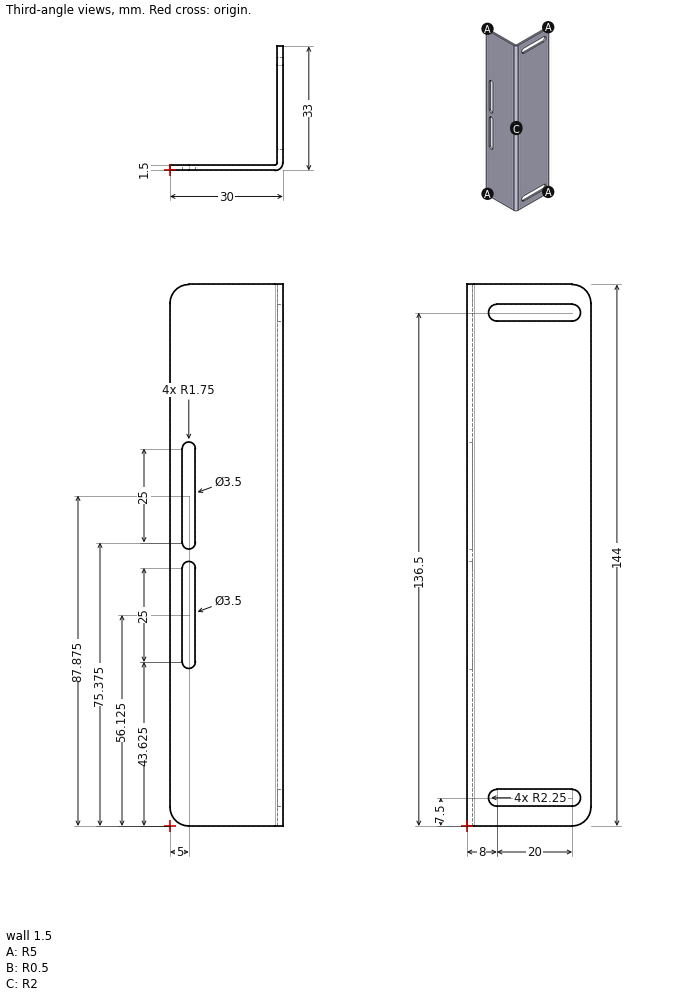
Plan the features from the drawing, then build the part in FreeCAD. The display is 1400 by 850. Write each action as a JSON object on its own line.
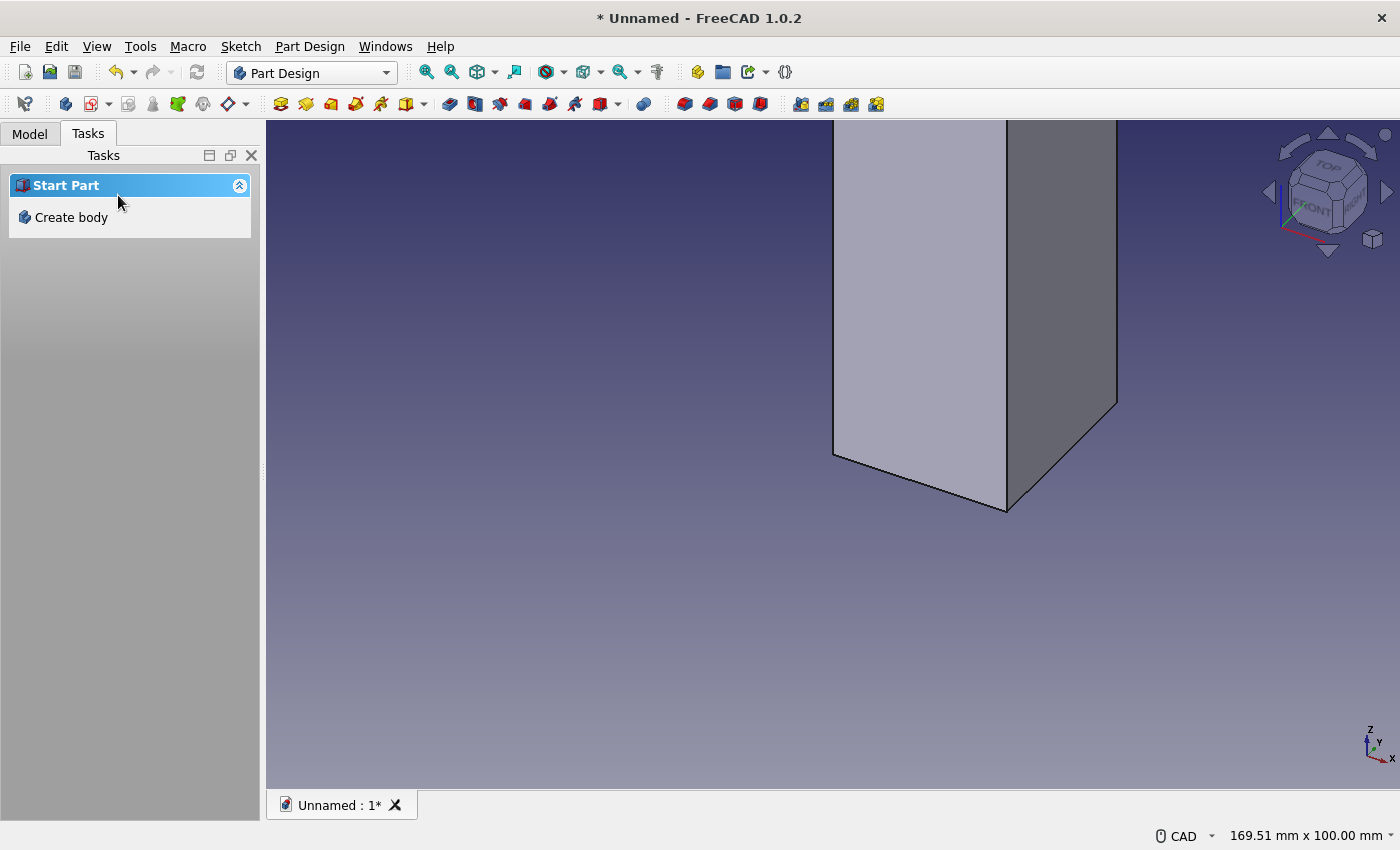
{"action": "left_click", "coordinate": [427, 72]}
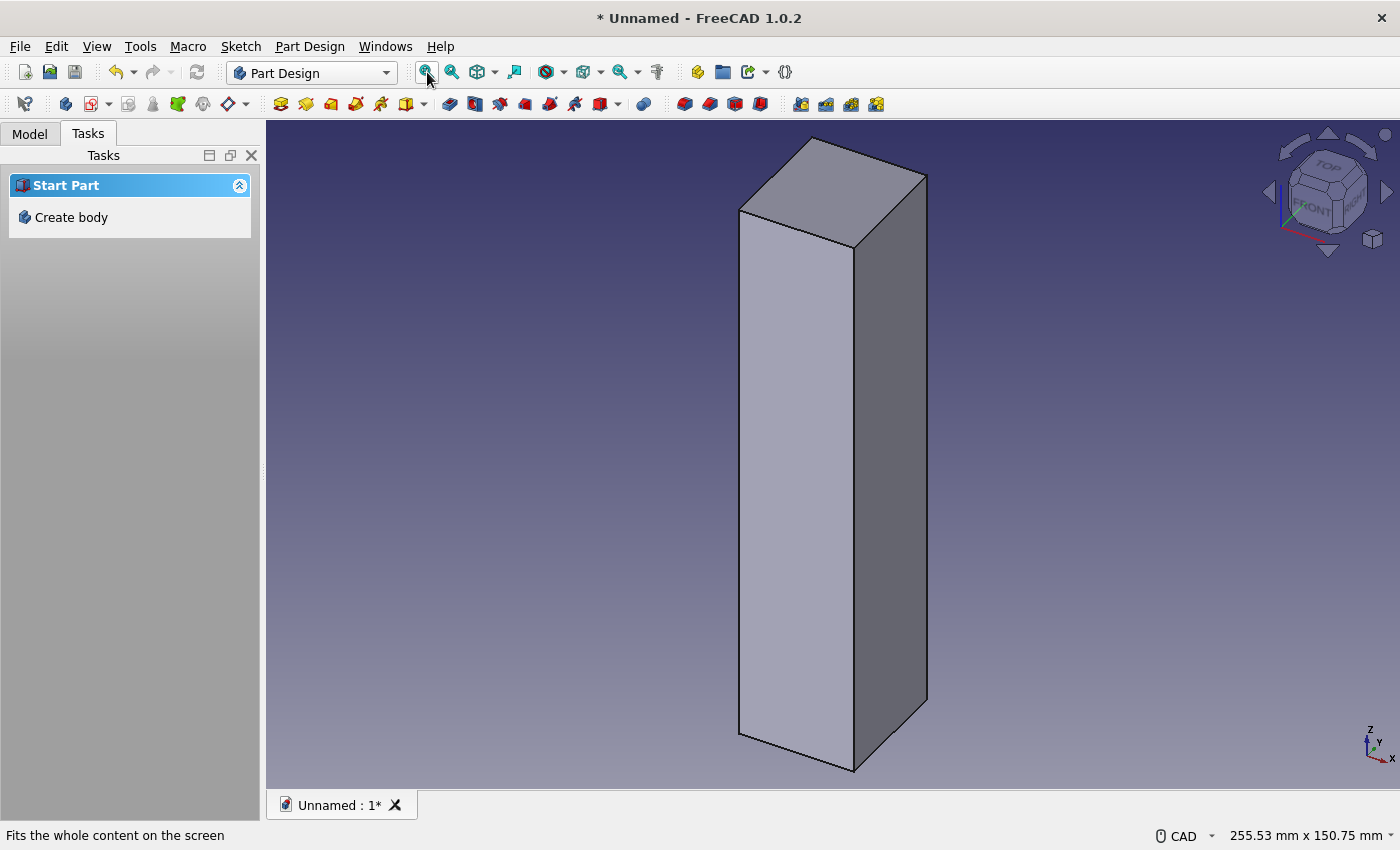
{"action": "left_click", "coordinate": [833, 192]}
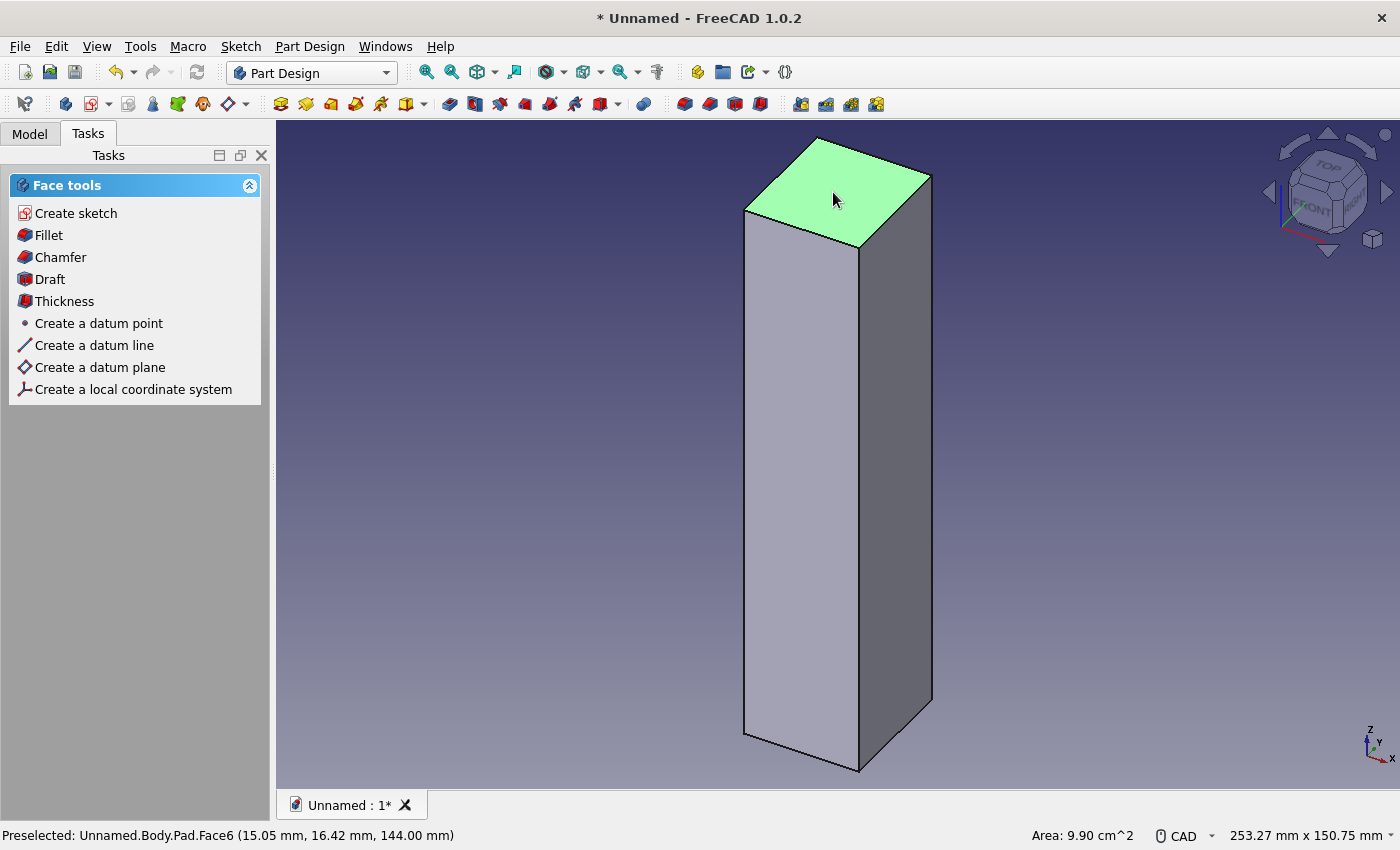
{"action": "key", "text": "0"}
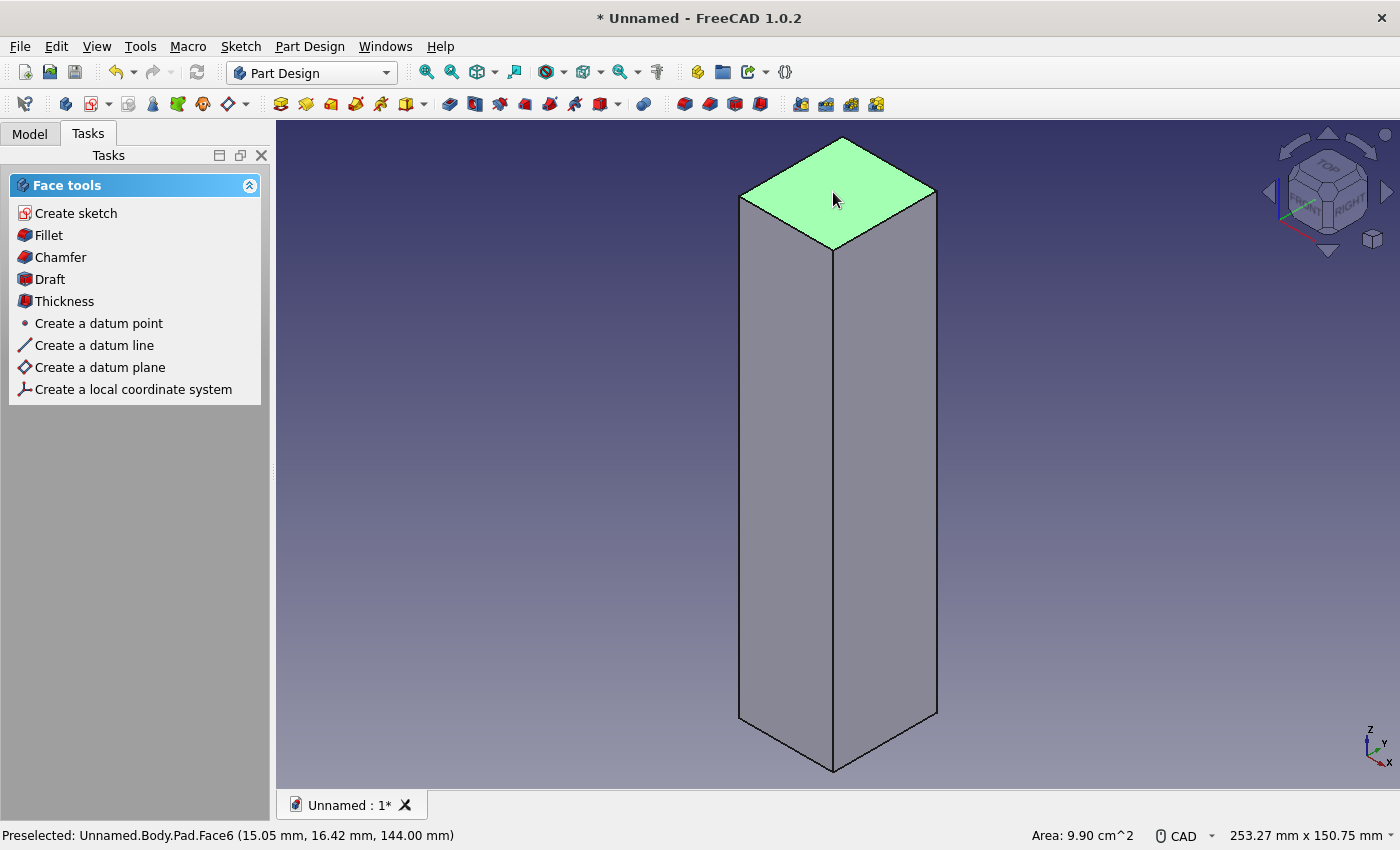
{"action": "key", "text": "2"}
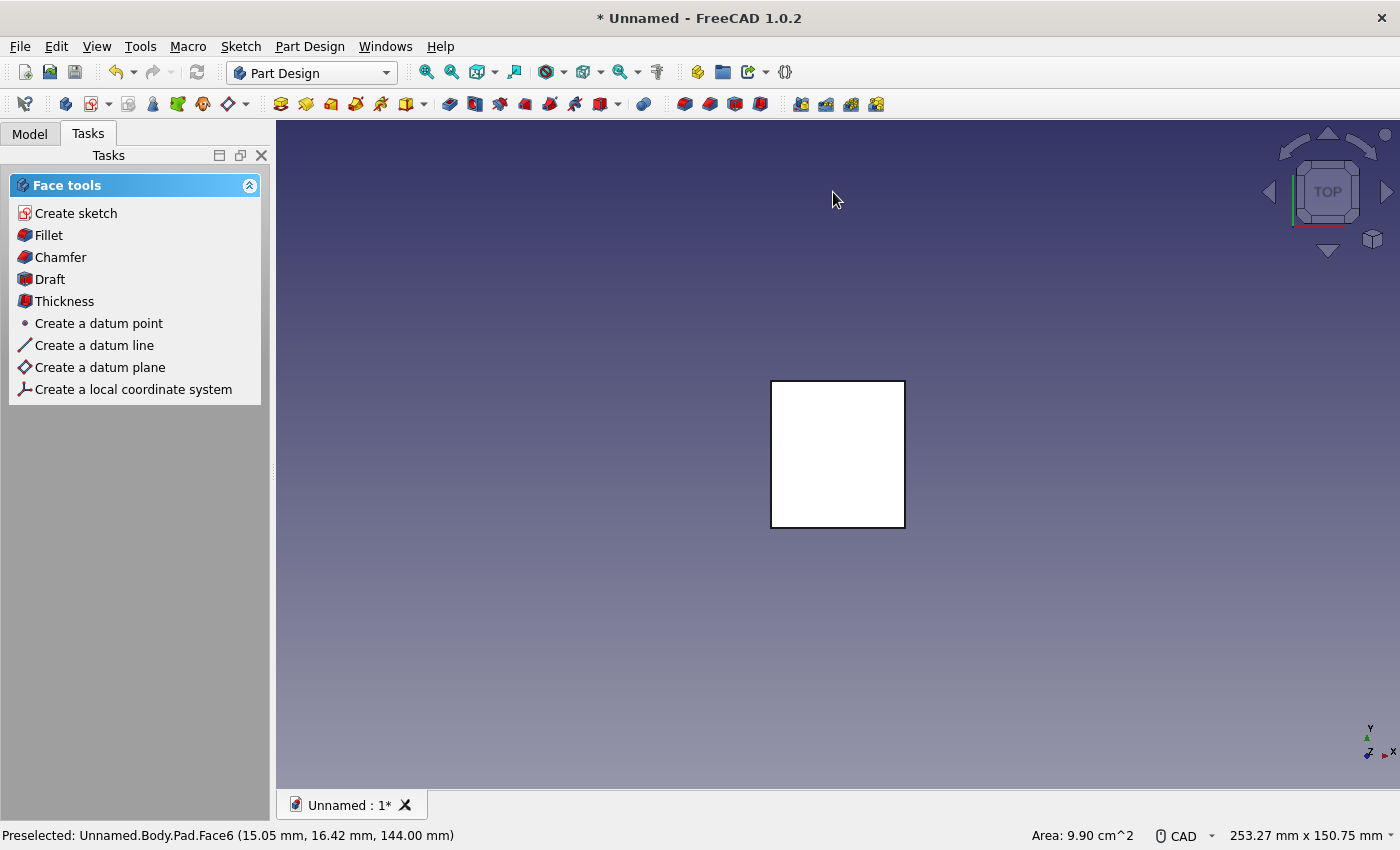
{"action": "left_click", "coordinate": [427, 72]}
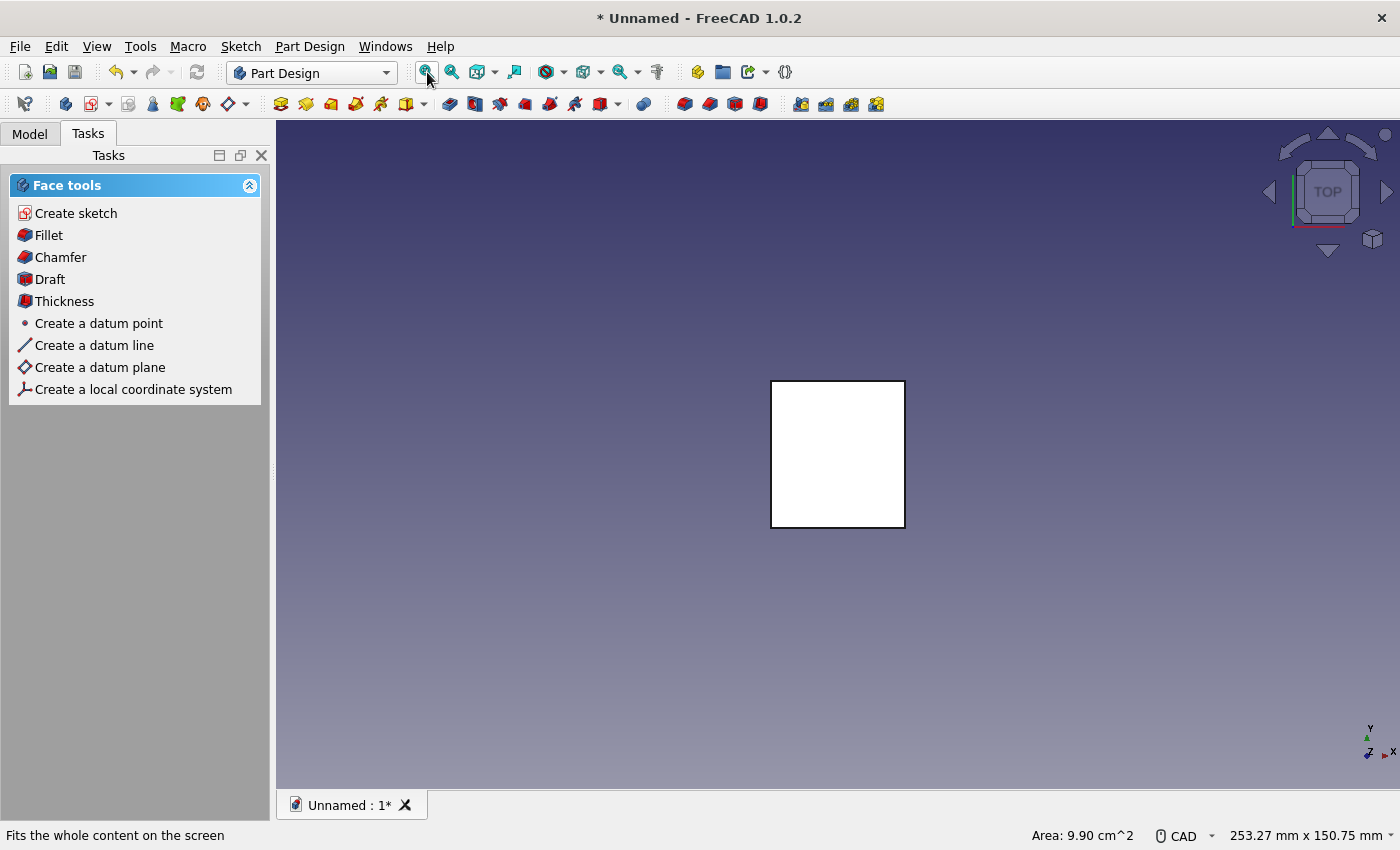
{"action": "key", "text": "1"}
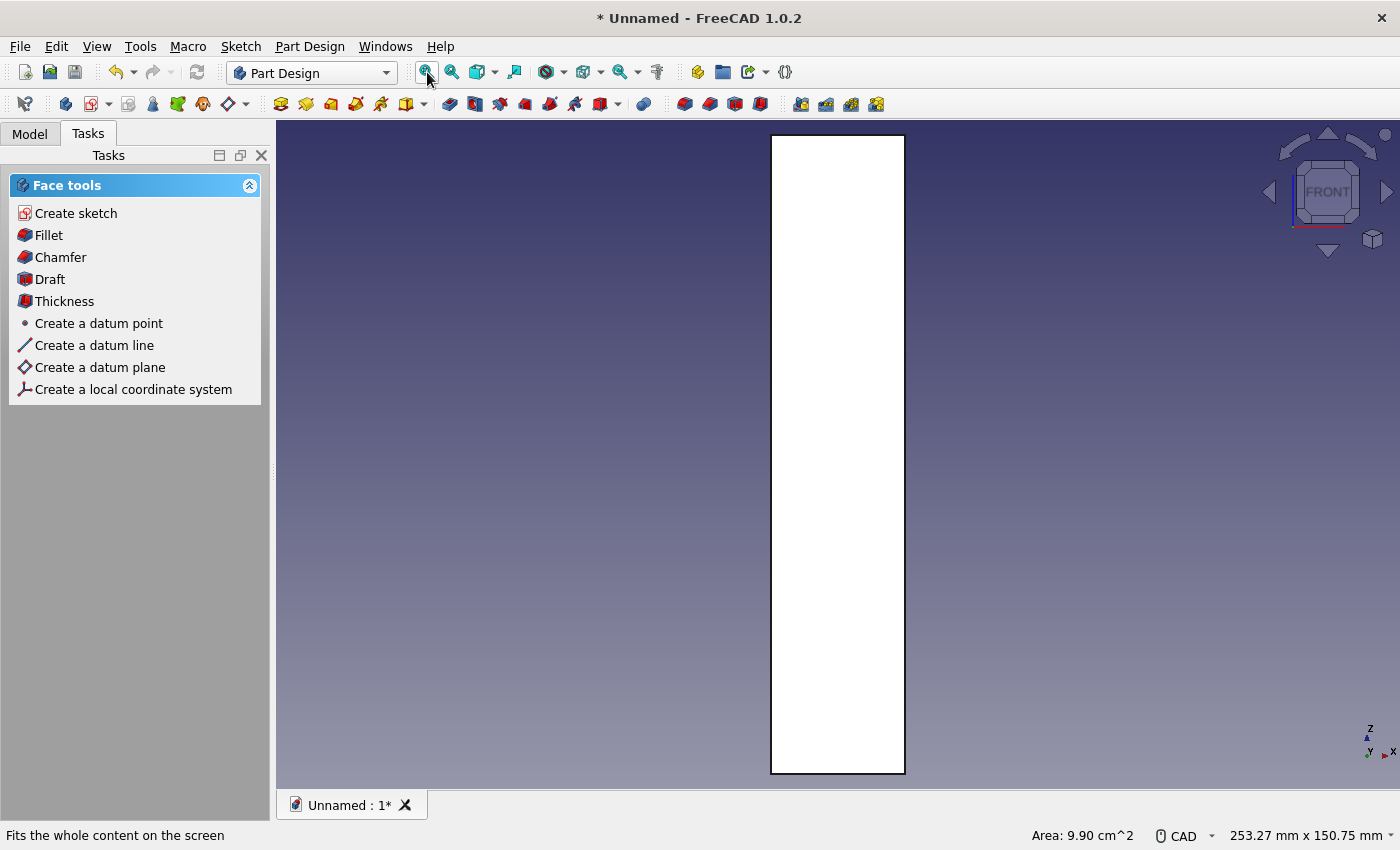
{"action": "key", "text": "3"}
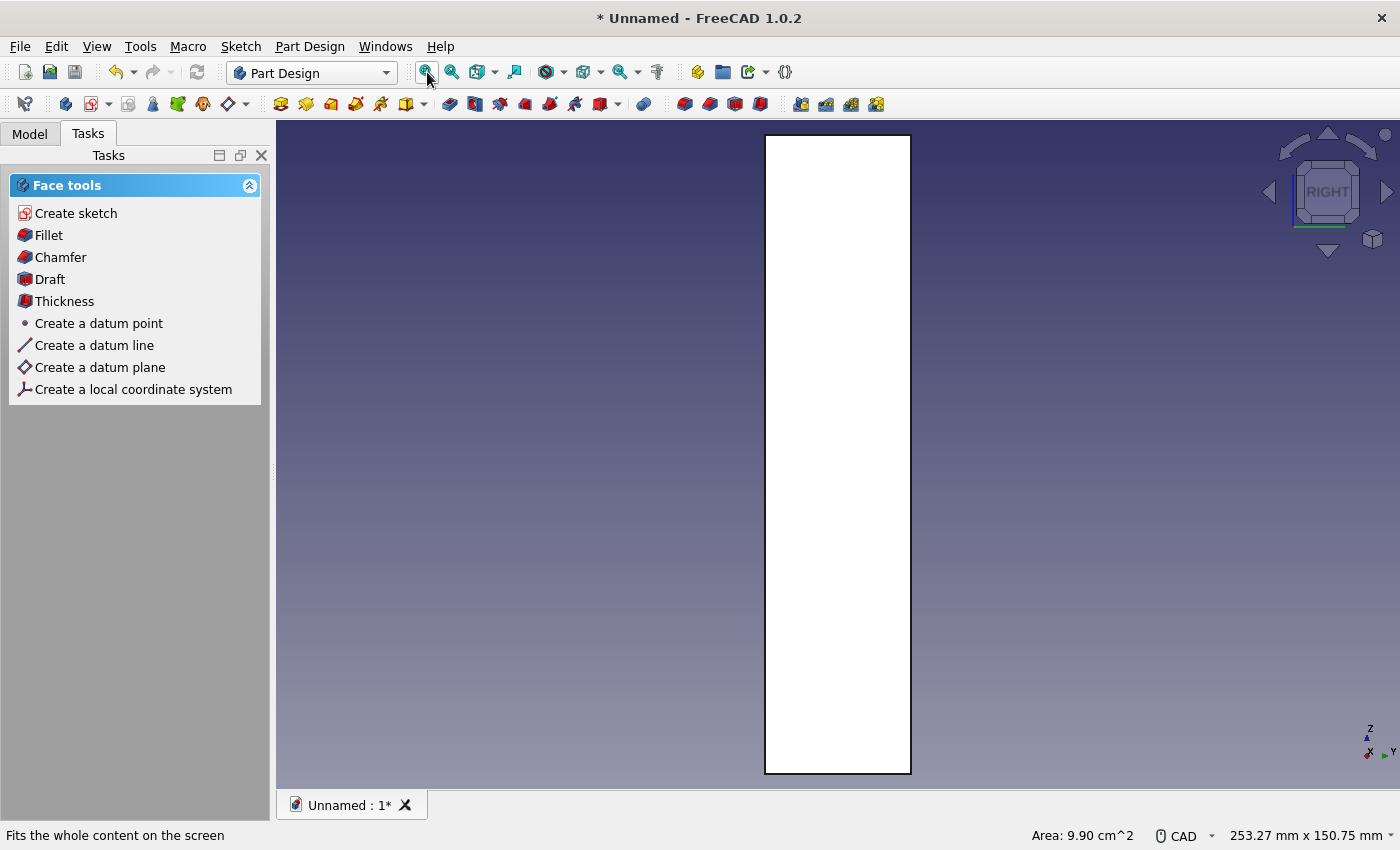
{"action": "key", "text": "5"}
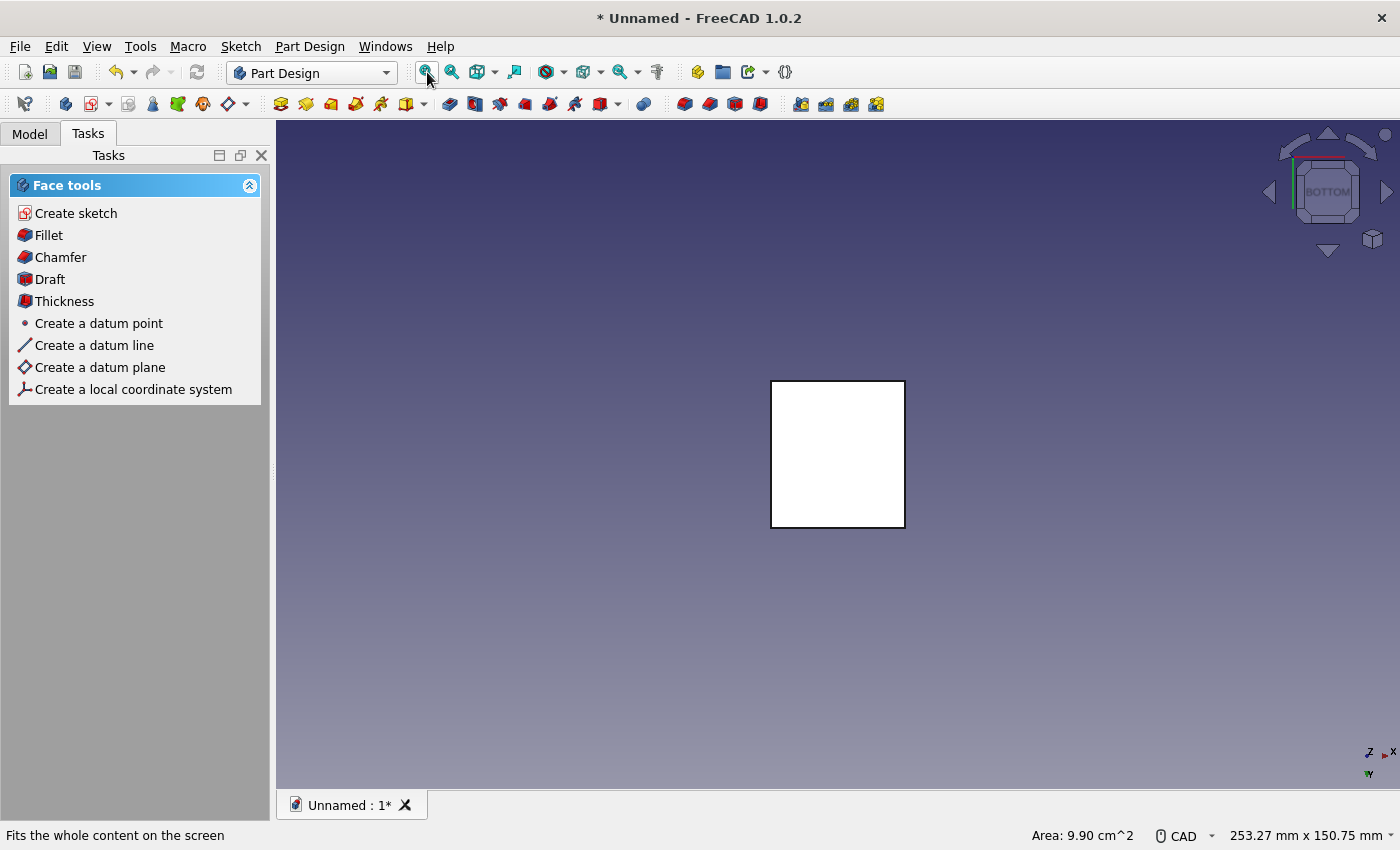
{"action": "left_click", "coordinate": [427, 72]}